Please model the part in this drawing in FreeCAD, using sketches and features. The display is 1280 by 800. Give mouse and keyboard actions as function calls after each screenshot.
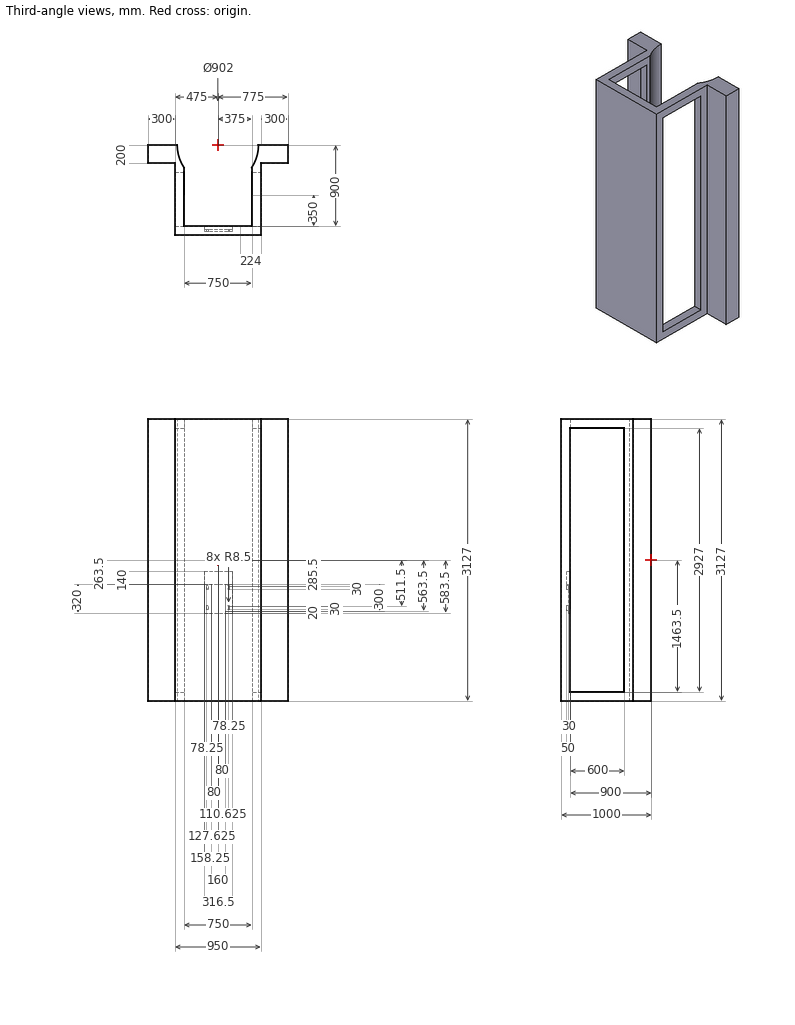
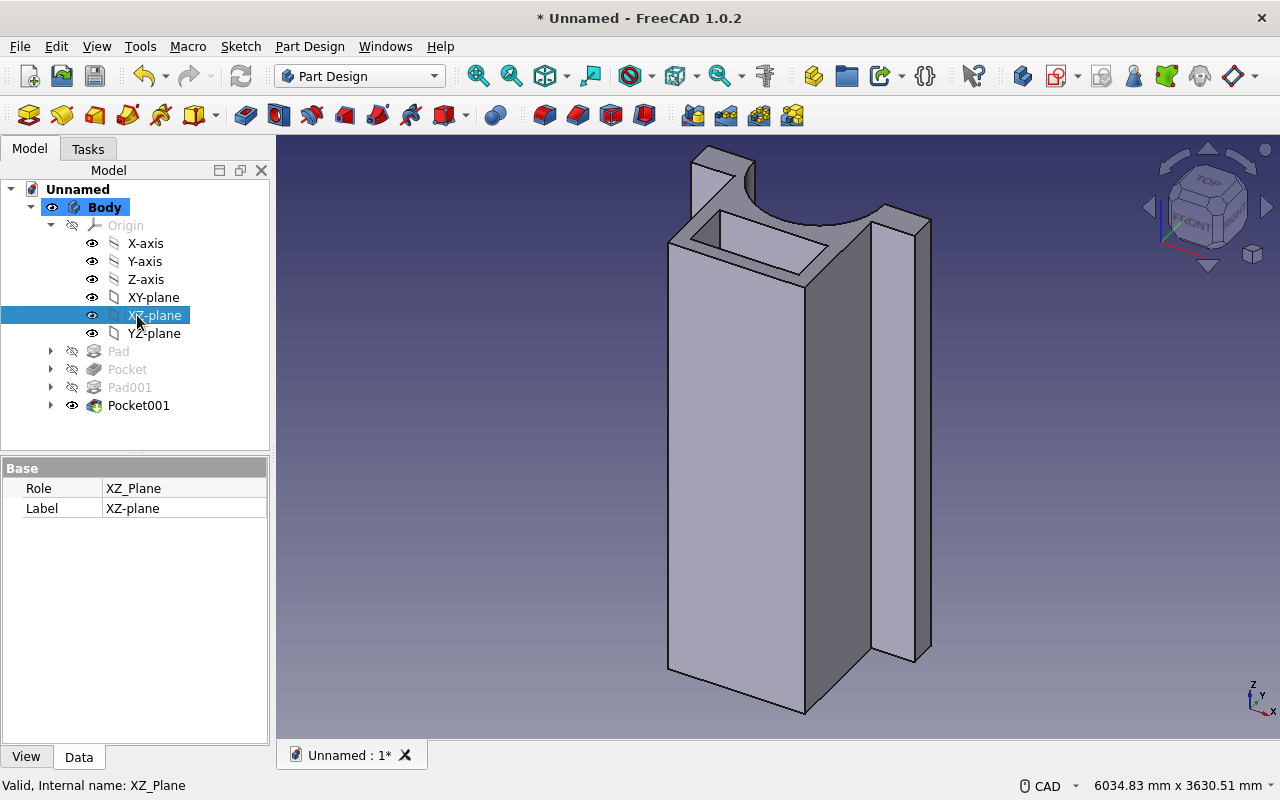
click(1232, 76)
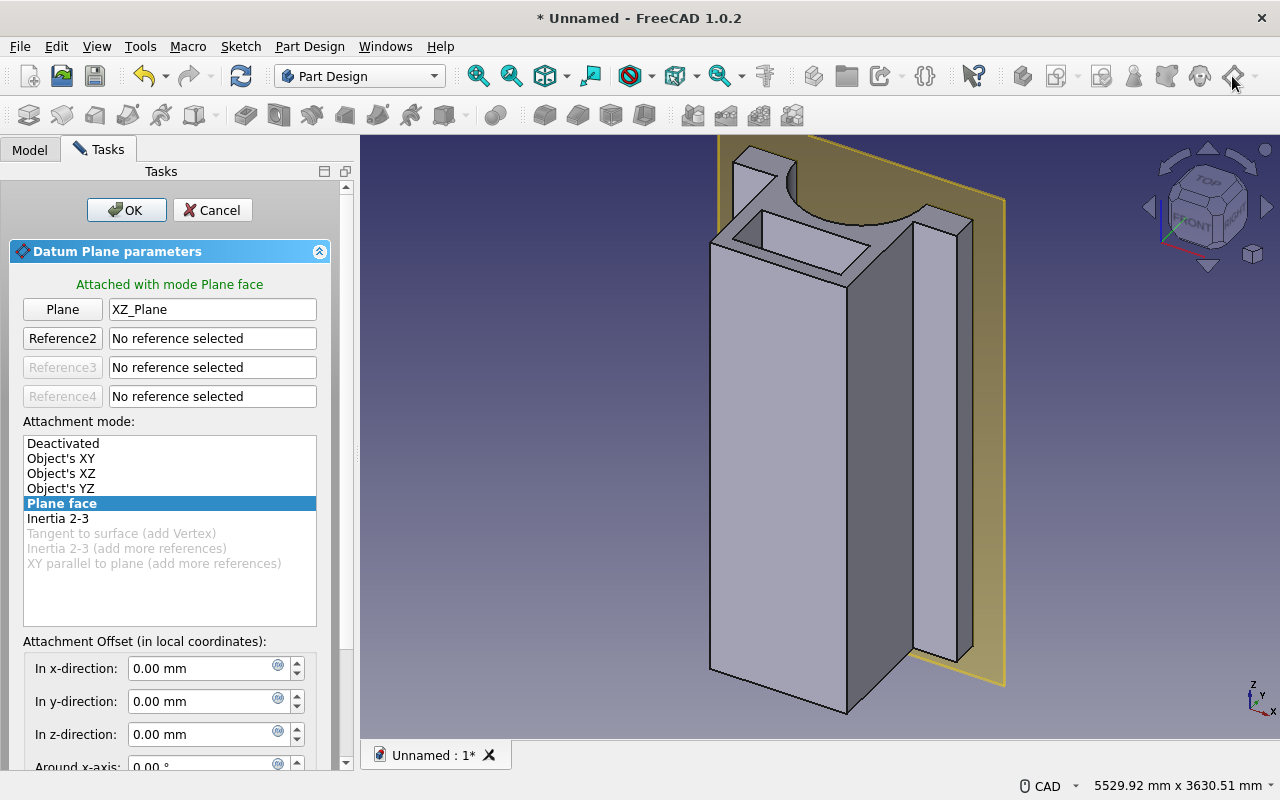
triple_click(210, 734)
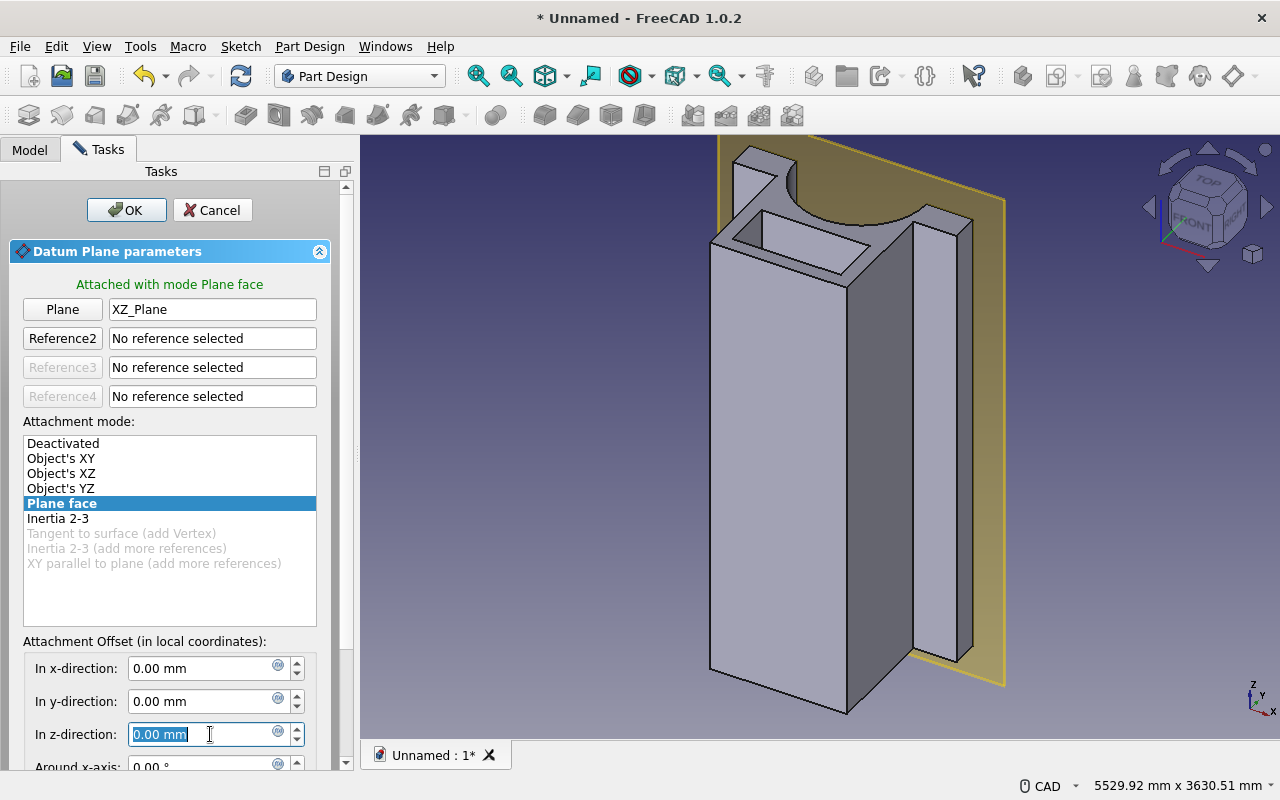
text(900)
key(Tab)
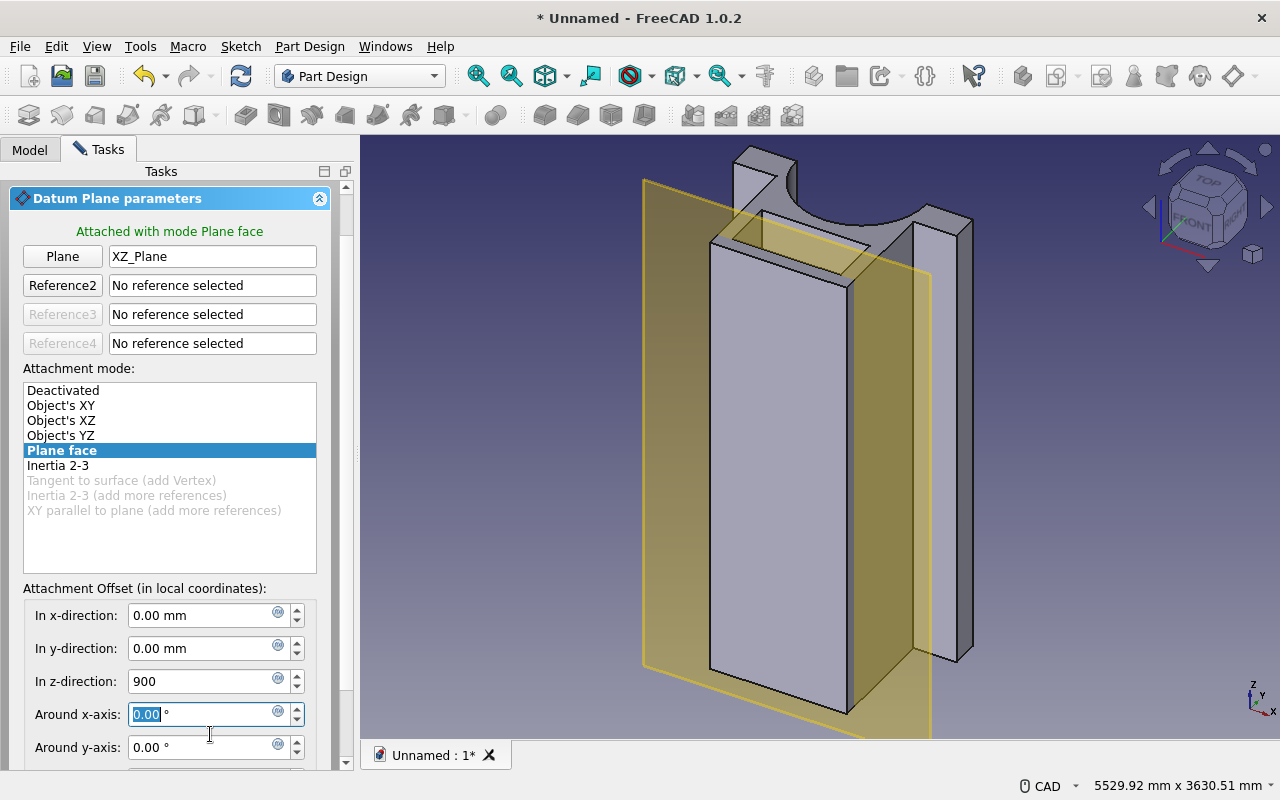
scroll(346, 476, up, 2)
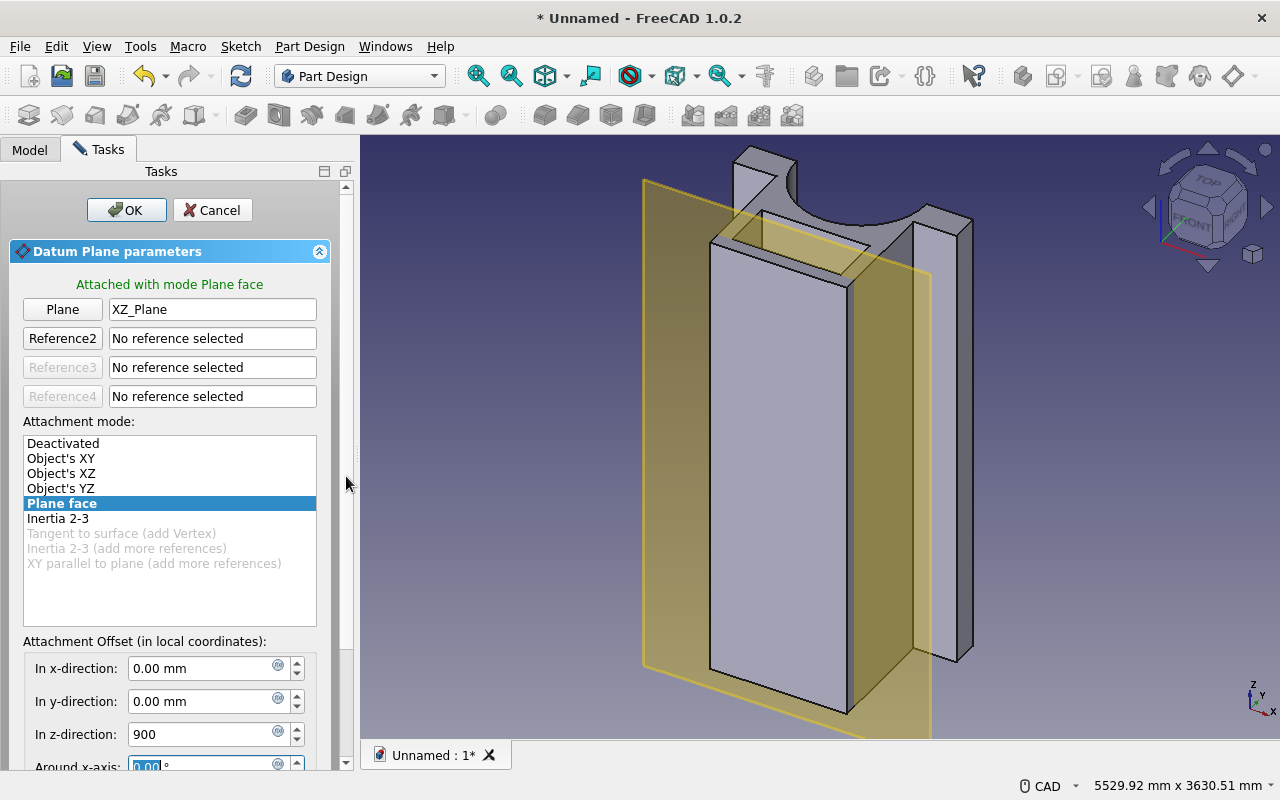
click(127, 210)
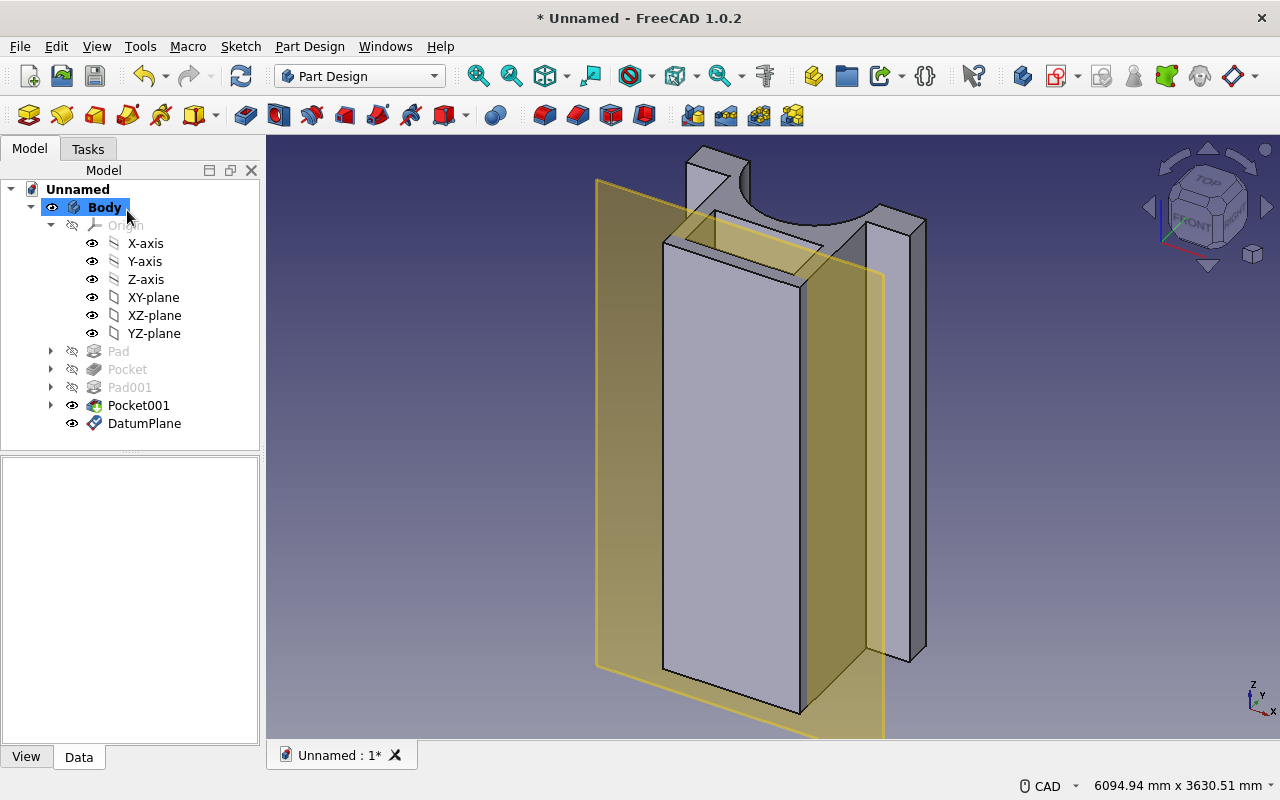
click(117, 423)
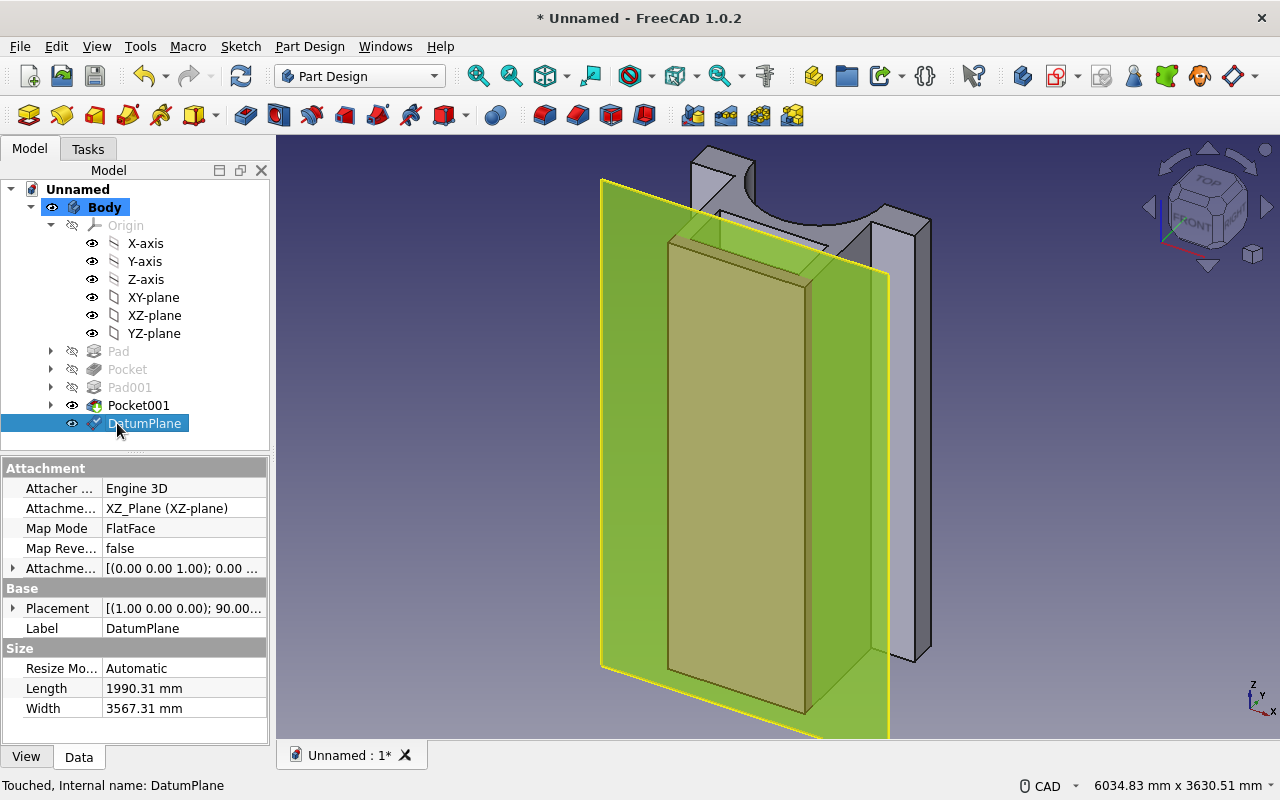
click(1056, 76)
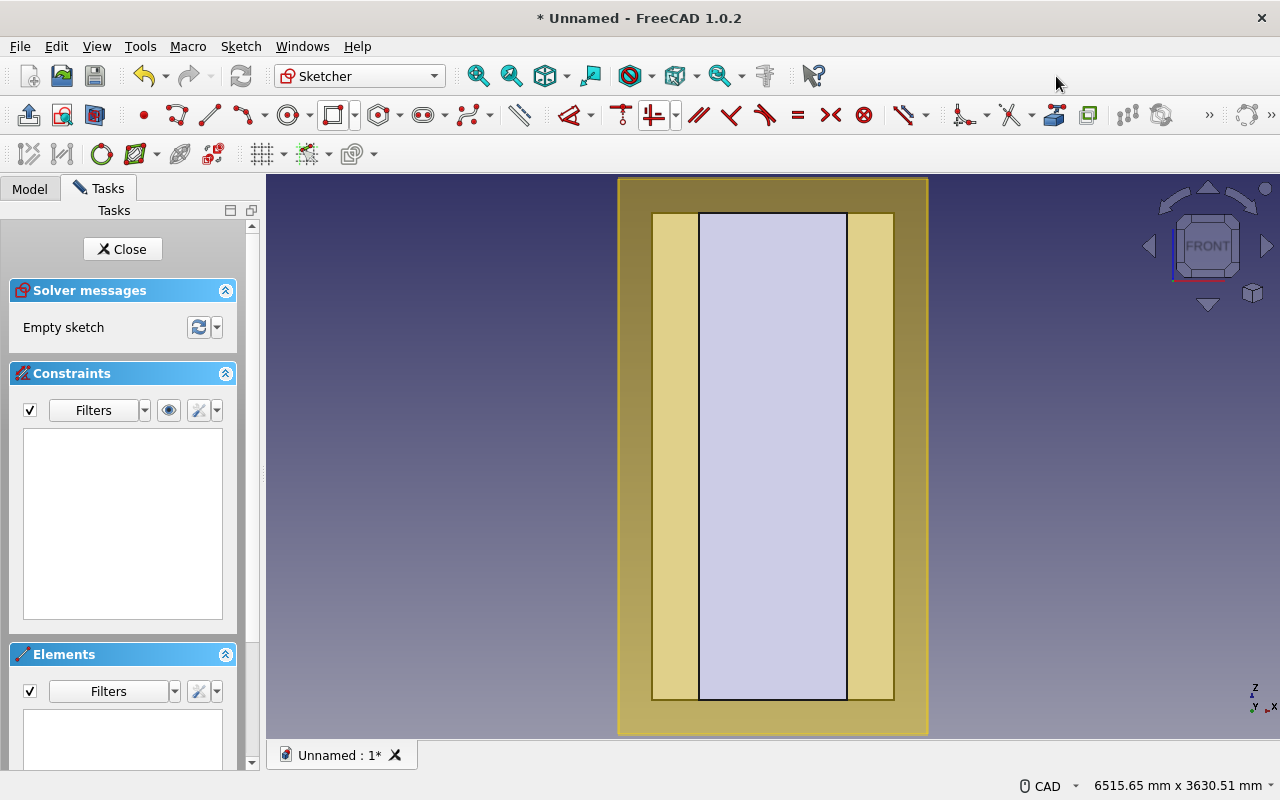
click(95, 116)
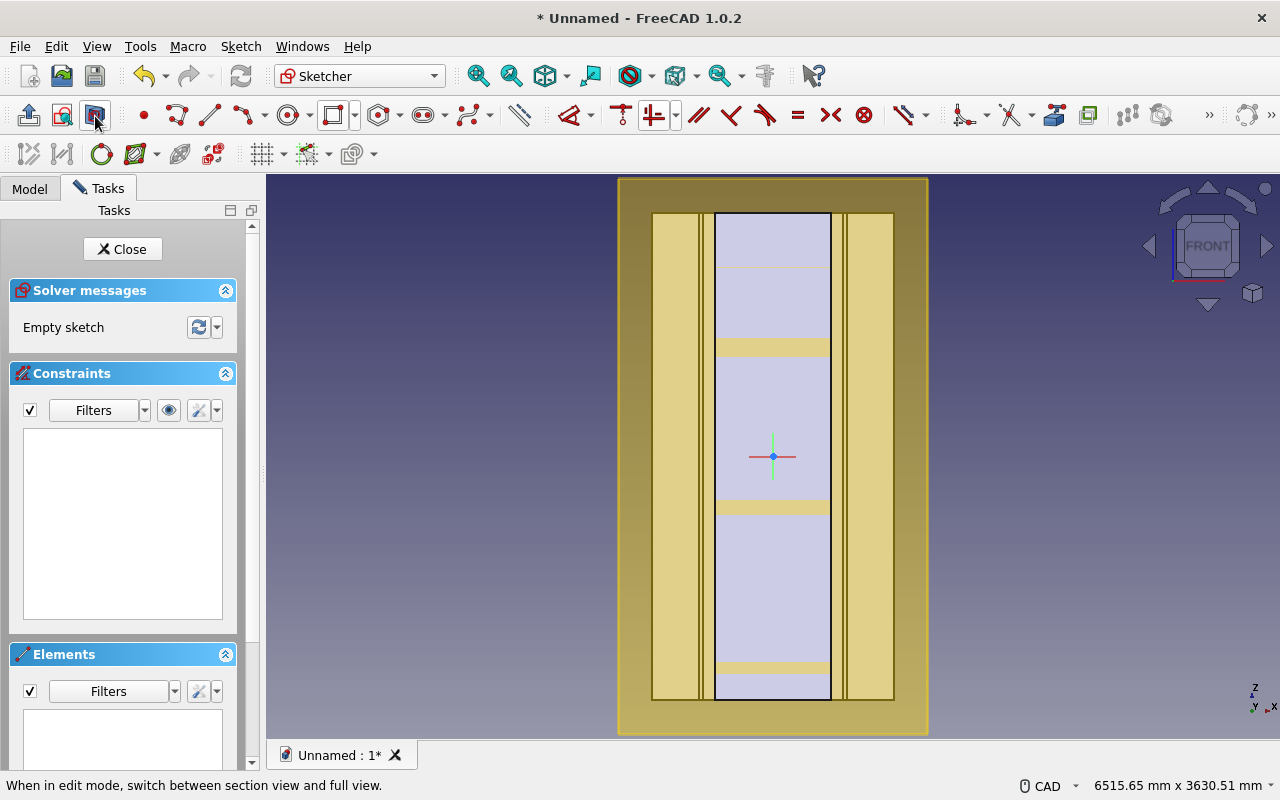
scroll(565, 457, down, 2)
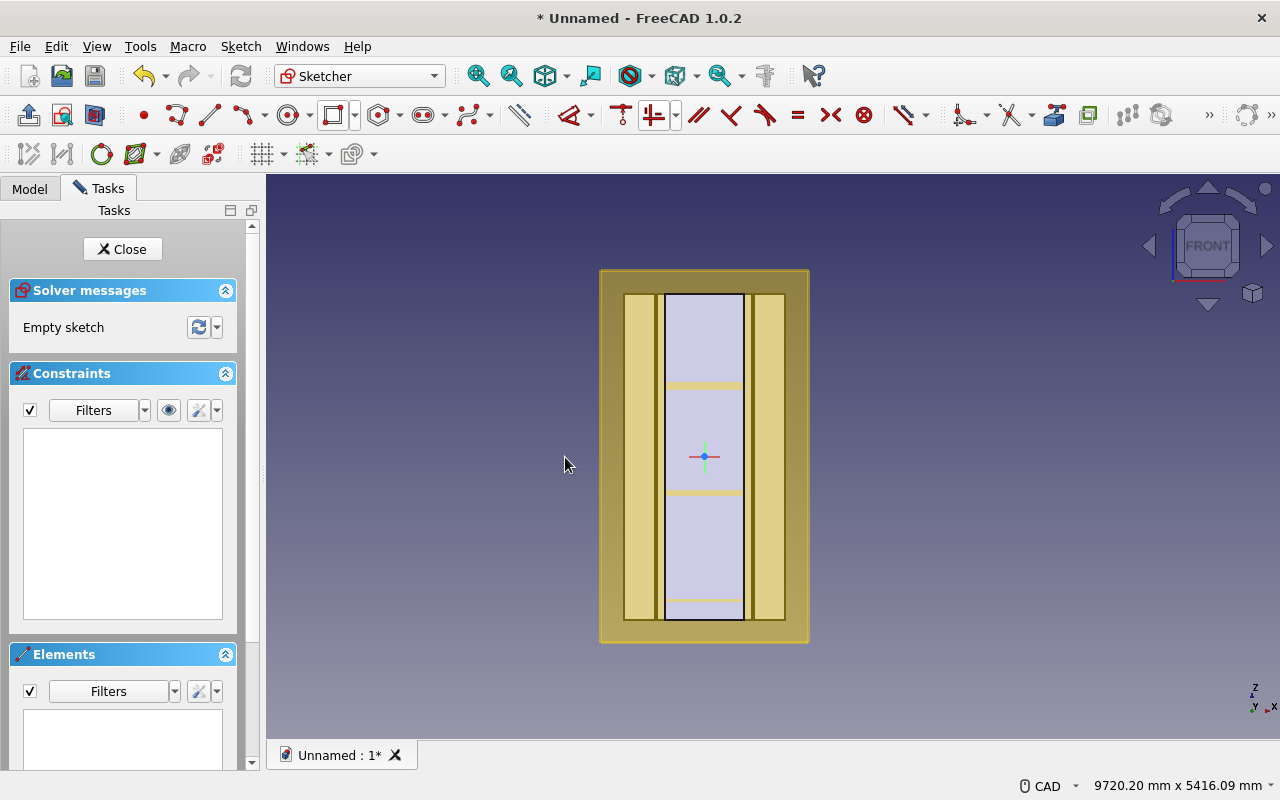
click(354, 116)